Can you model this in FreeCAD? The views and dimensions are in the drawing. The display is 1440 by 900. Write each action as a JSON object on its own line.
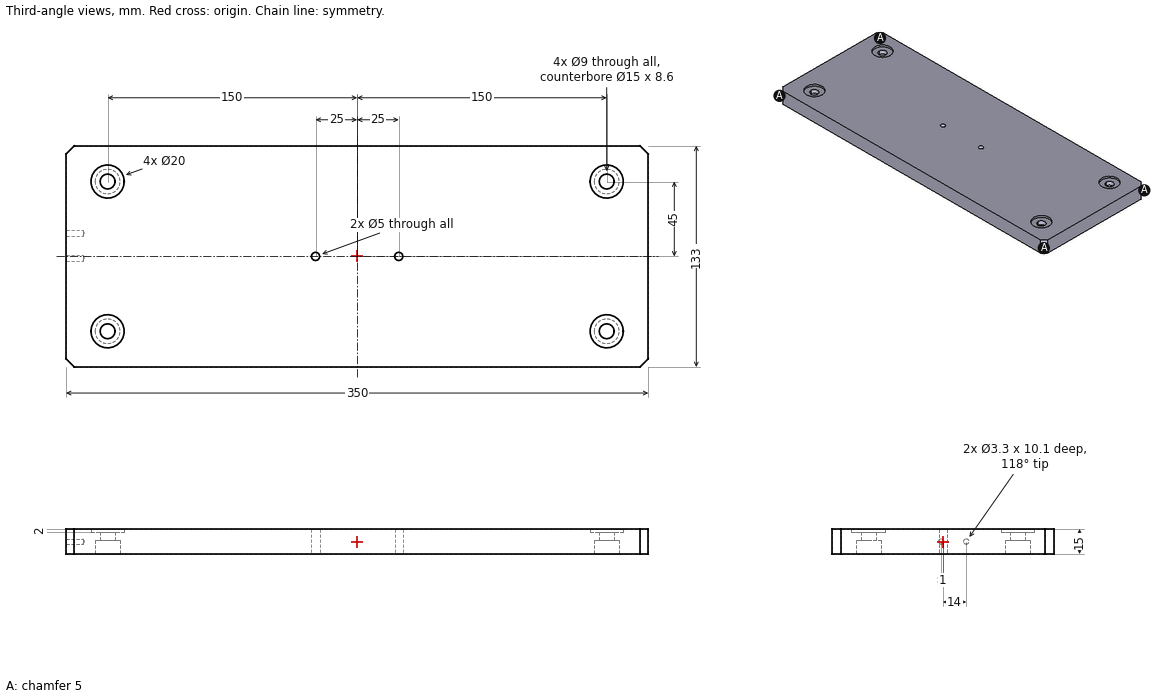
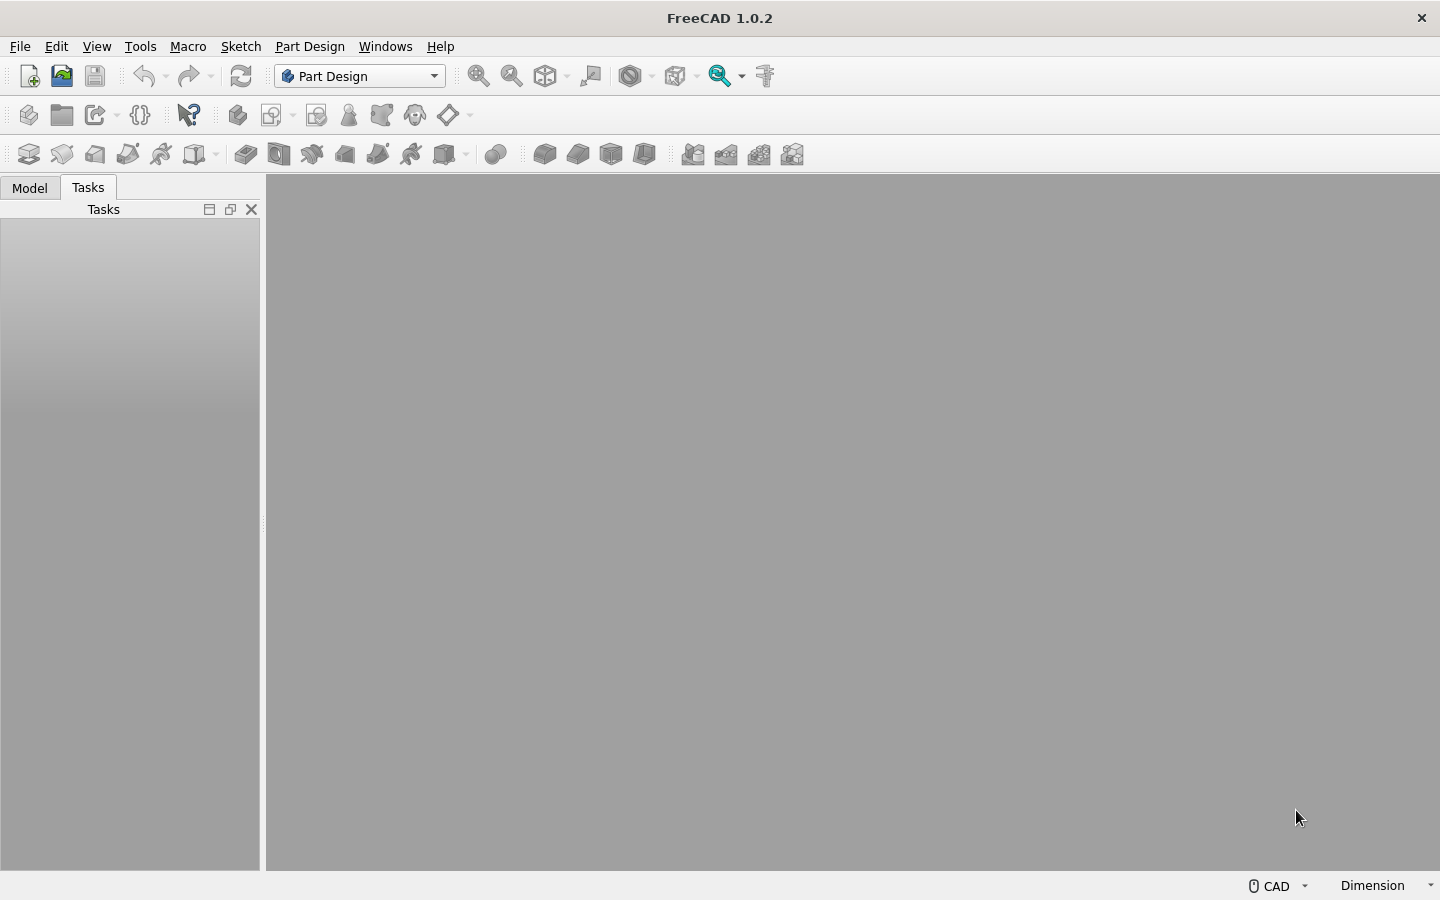
{"action": "left_click", "coordinate": [29, 76]}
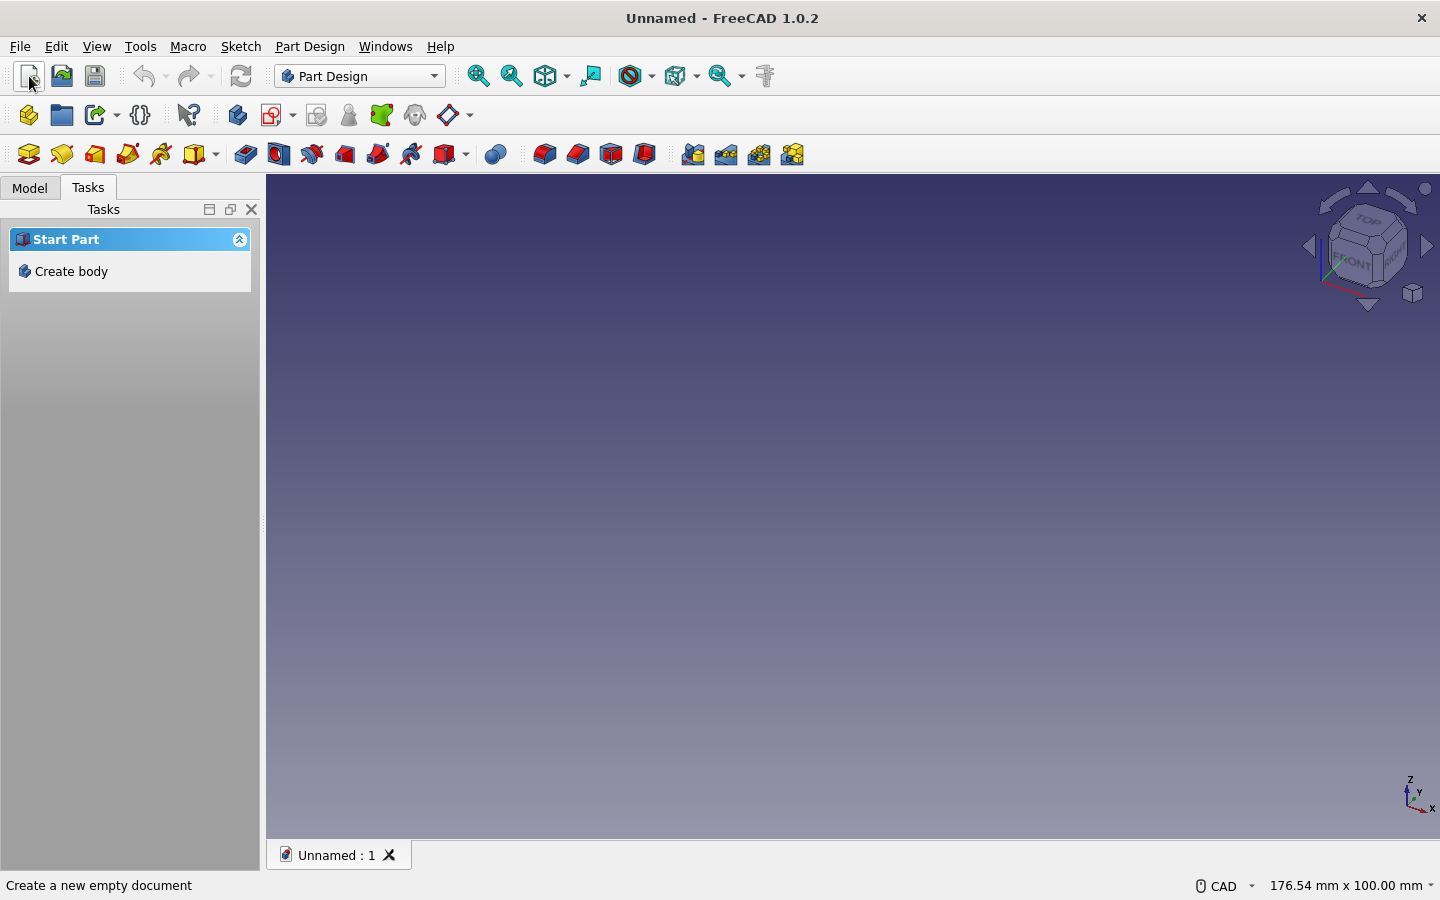
{"action": "left_click", "coordinate": [270, 116]}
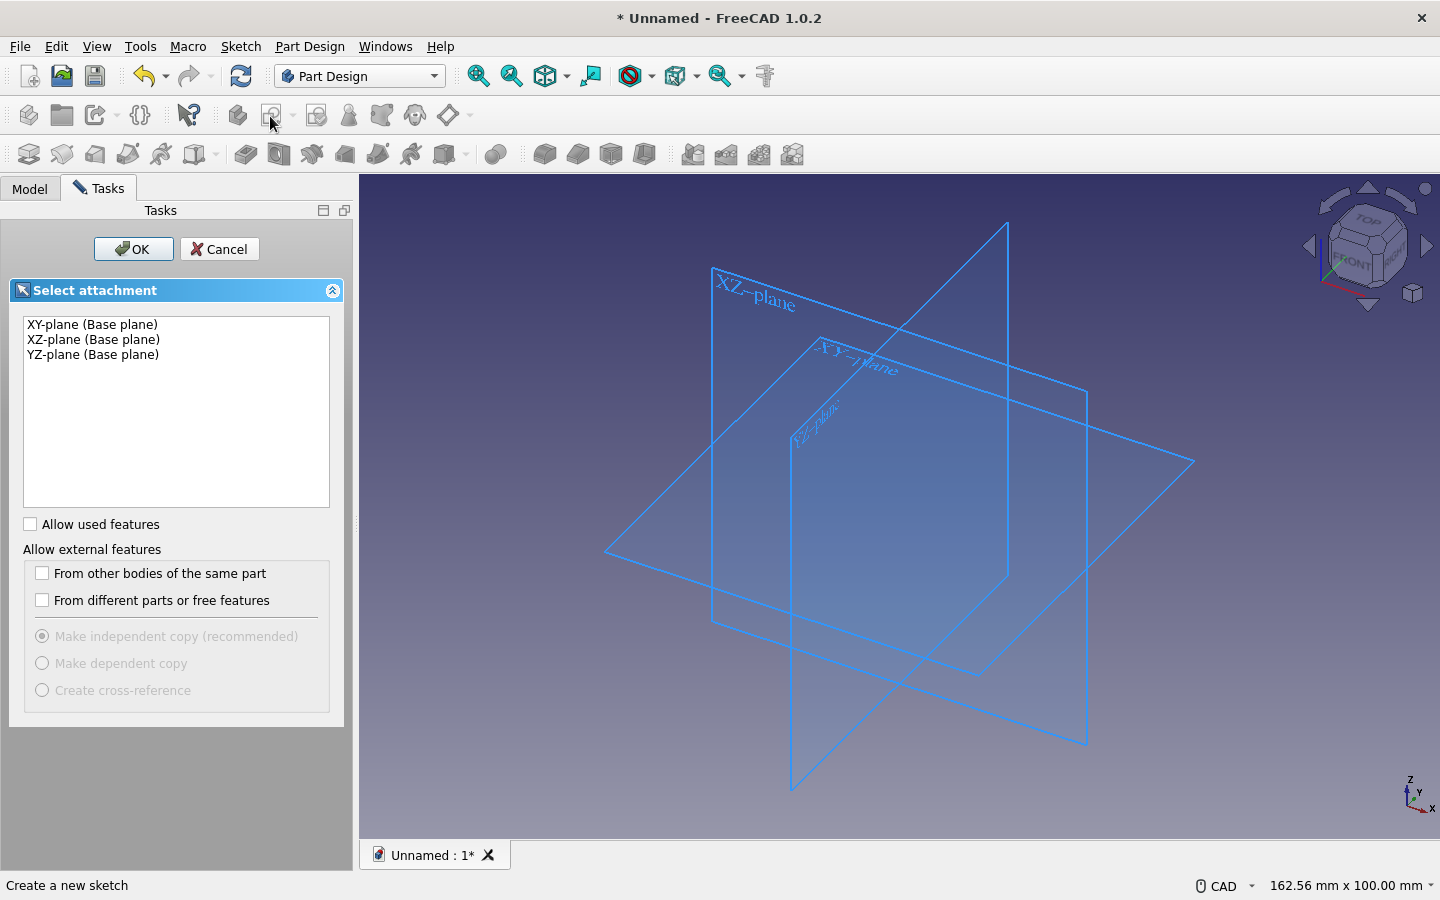
{"action": "left_click", "coordinate": [84, 324]}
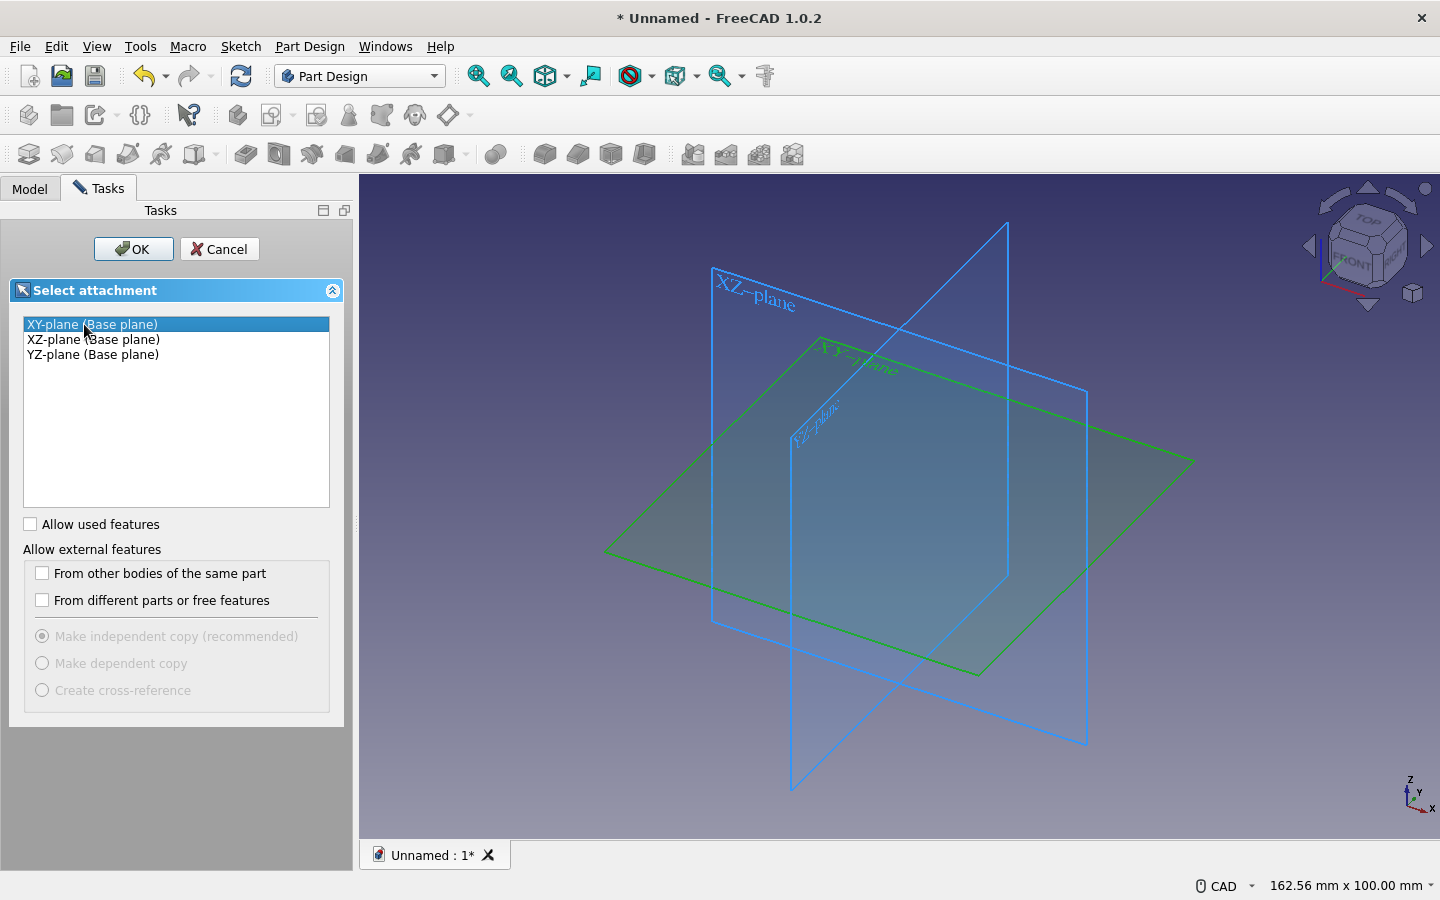
{"action": "left_click", "coordinate": [134, 249]}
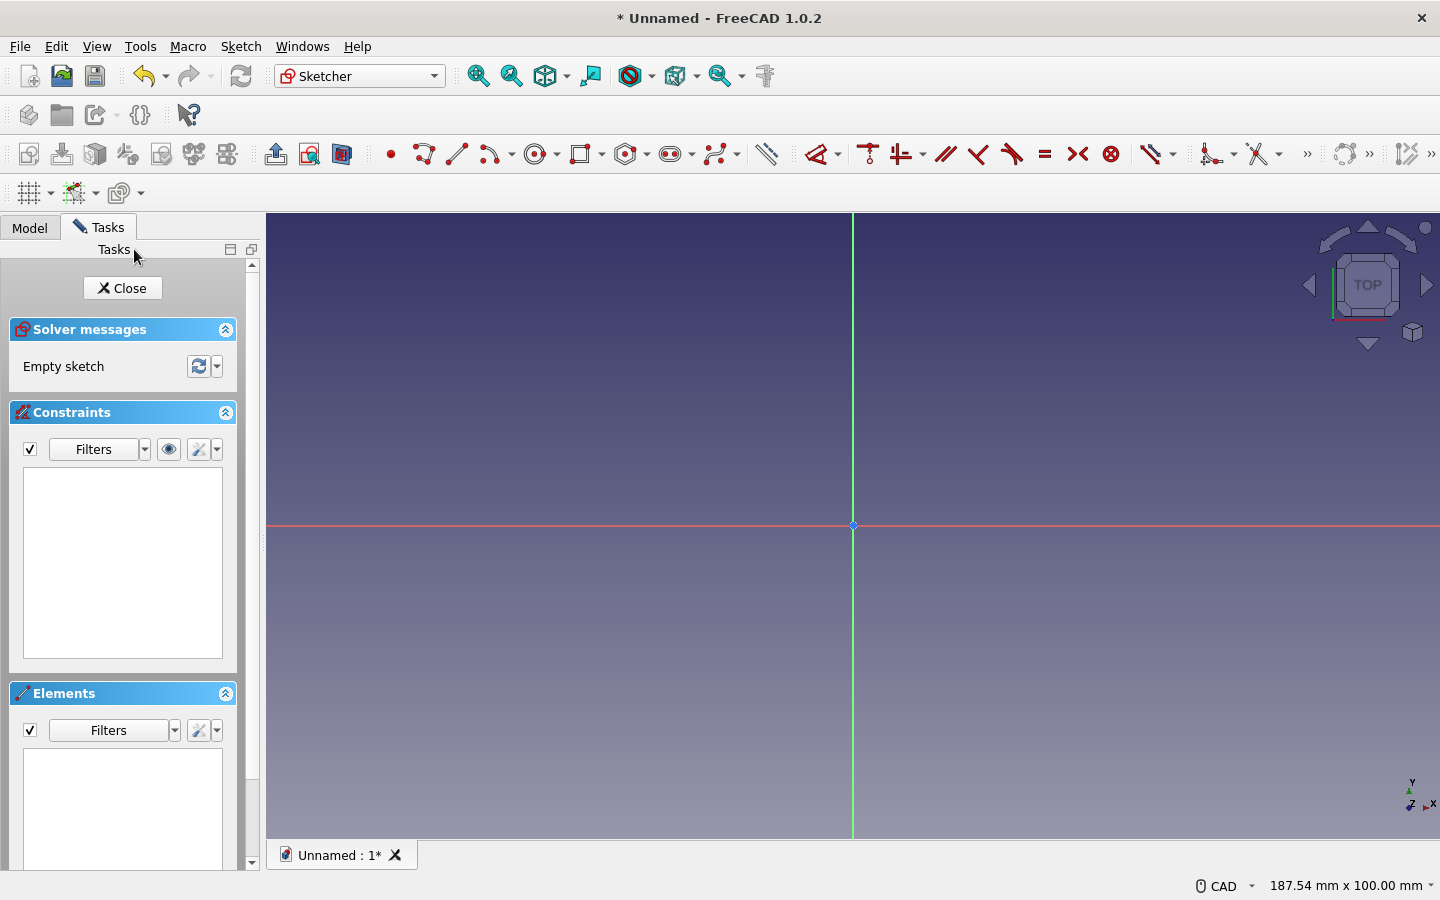
{"action": "scroll", "coordinate": [755, 526], "scroll_direction": "down", "scroll_amount": 6}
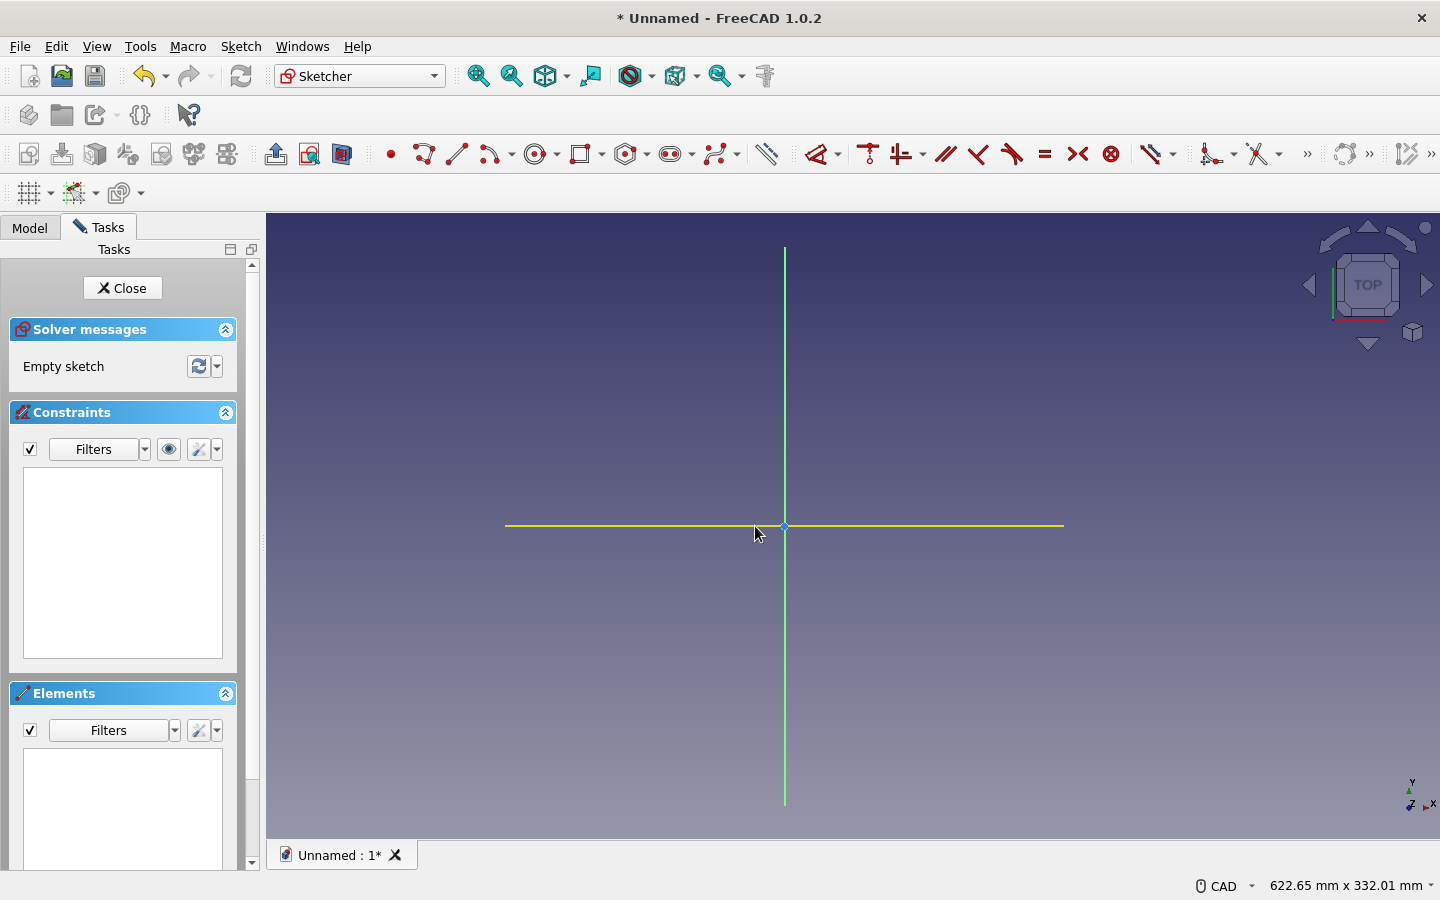
{"action": "key", "text": "g v"}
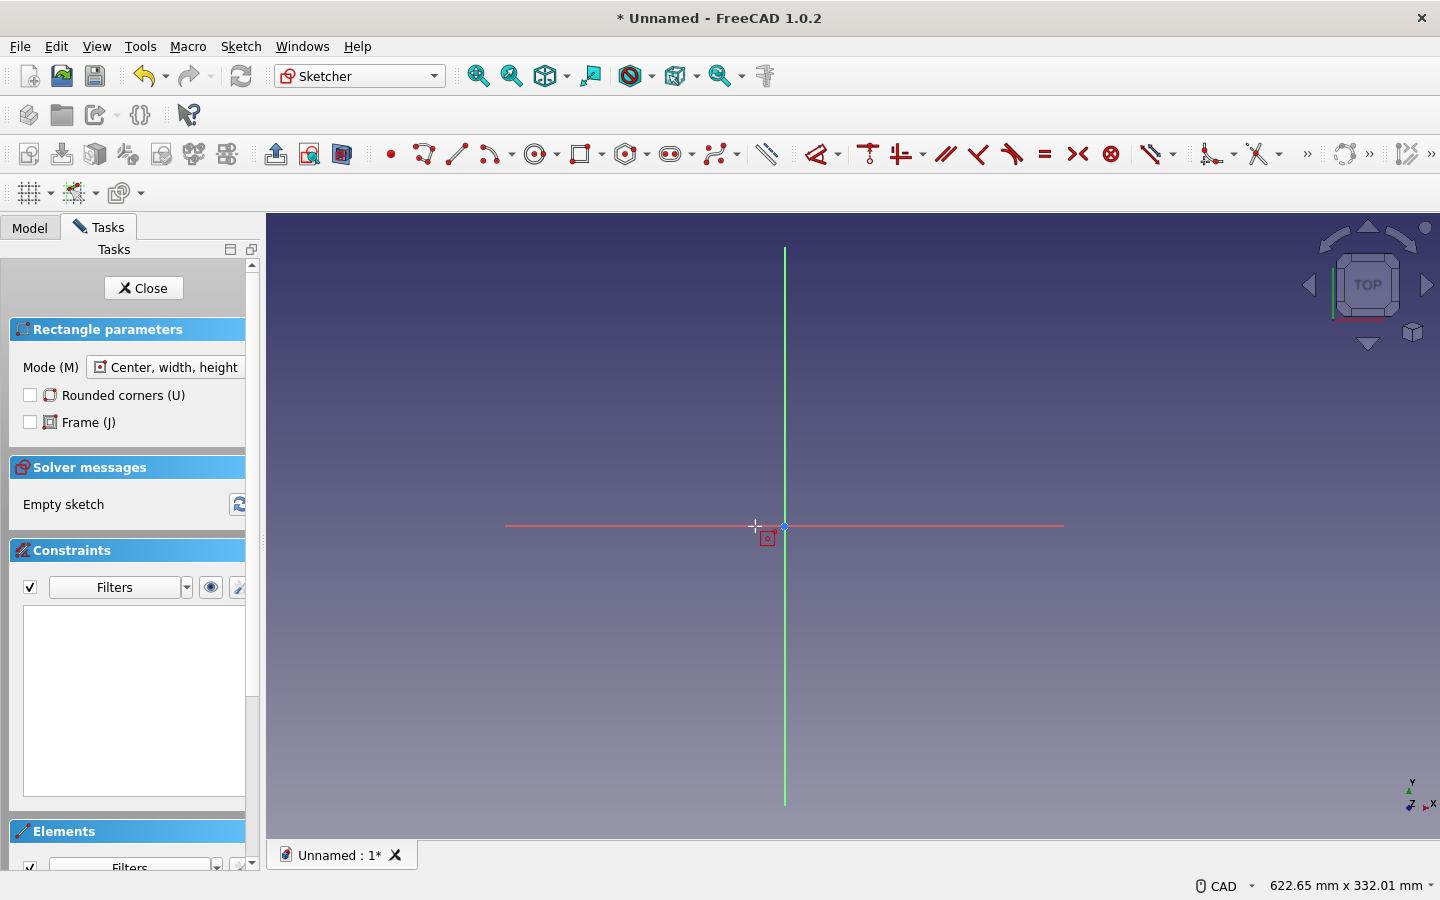
{"action": "left_click", "coordinate": [785, 526]}
{"action": "mouse_move", "coordinate": [1115, 401]}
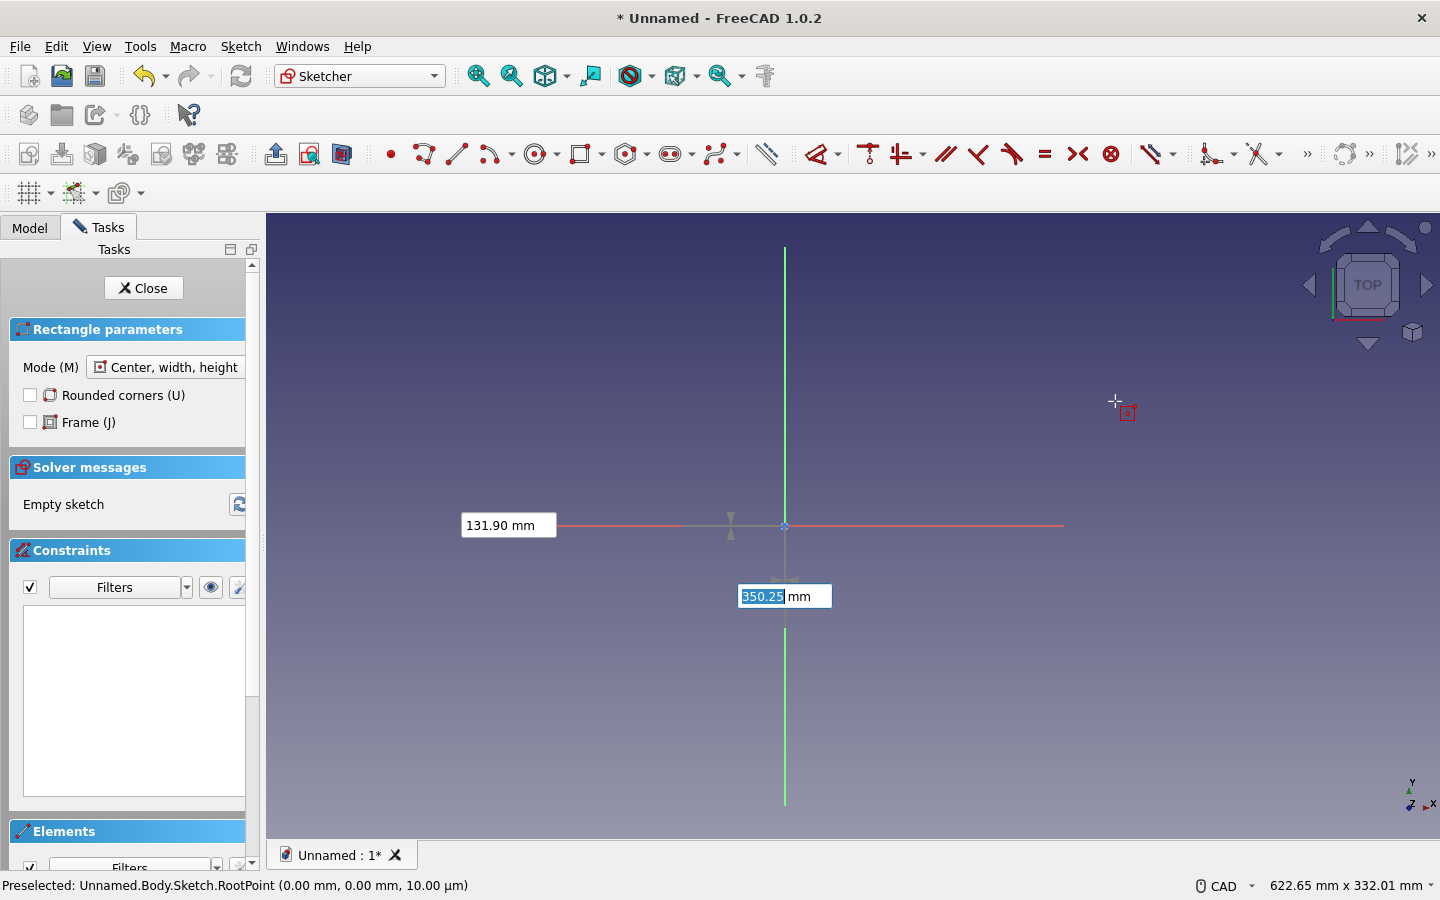
{"action": "type", "text": "350"}
{"action": "key", "text": "Tab"}
{"action": "type", "text": "133"}
{"action": "key", "text": "Return"}
{"action": "key", "text": "Escape"}